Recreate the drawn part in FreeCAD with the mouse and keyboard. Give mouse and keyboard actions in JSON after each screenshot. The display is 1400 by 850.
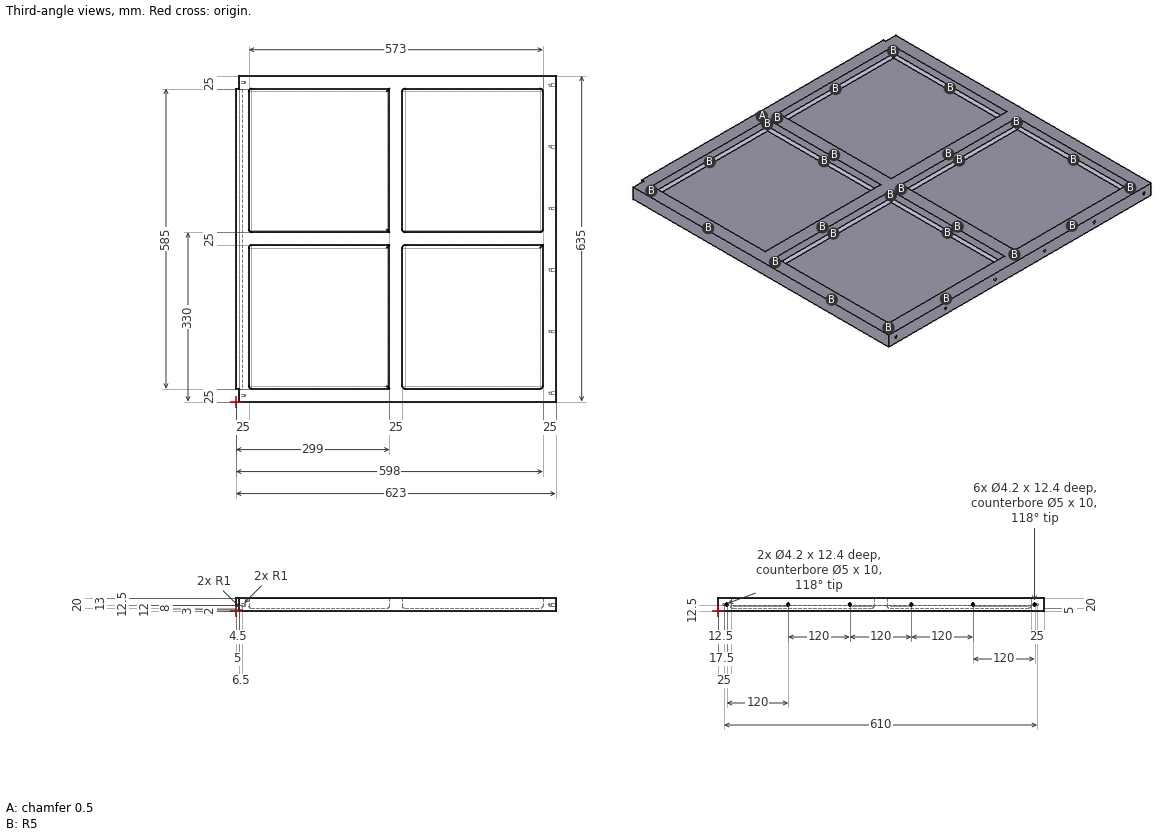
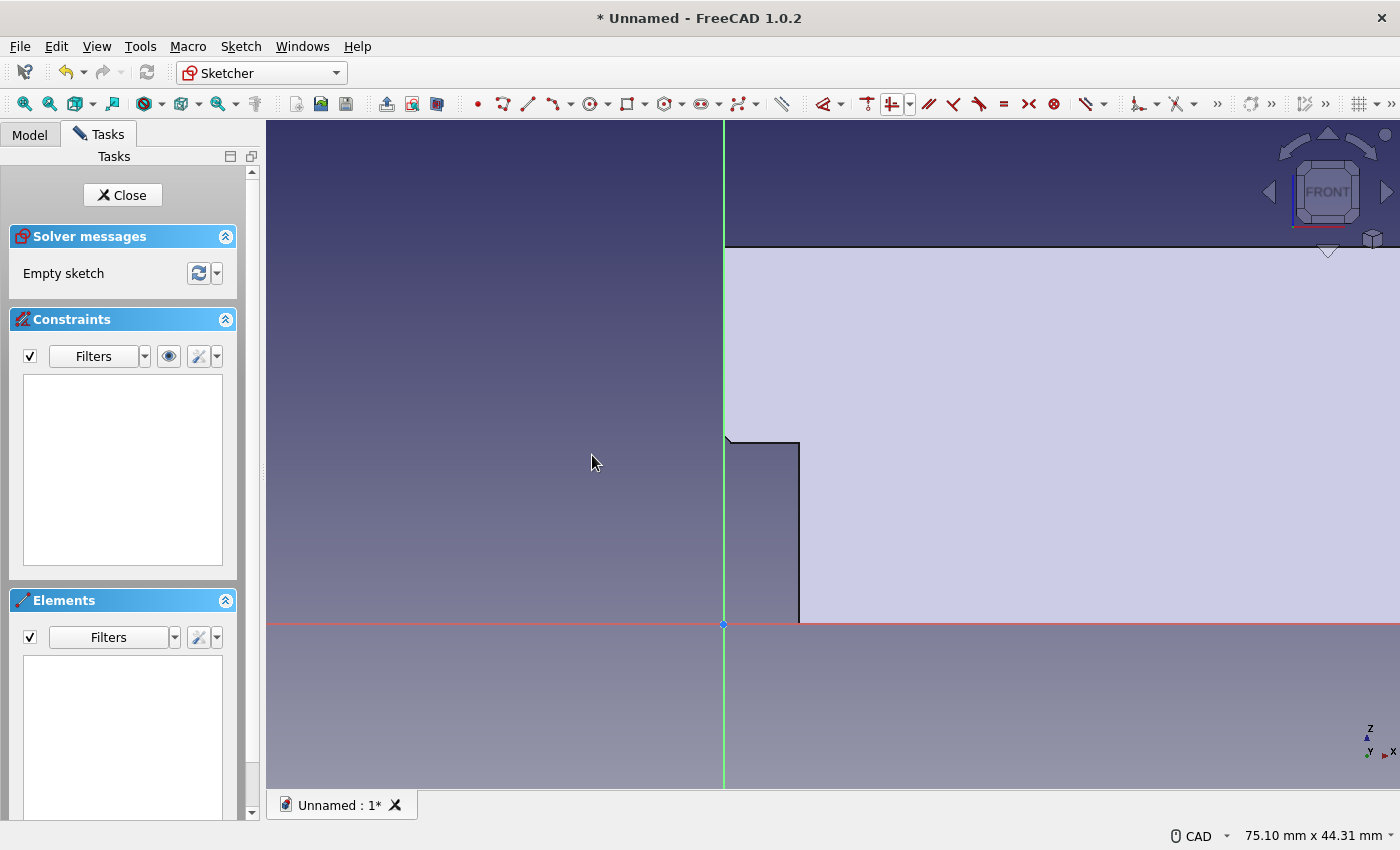
{"action": "left_click", "coordinate": [503, 104]}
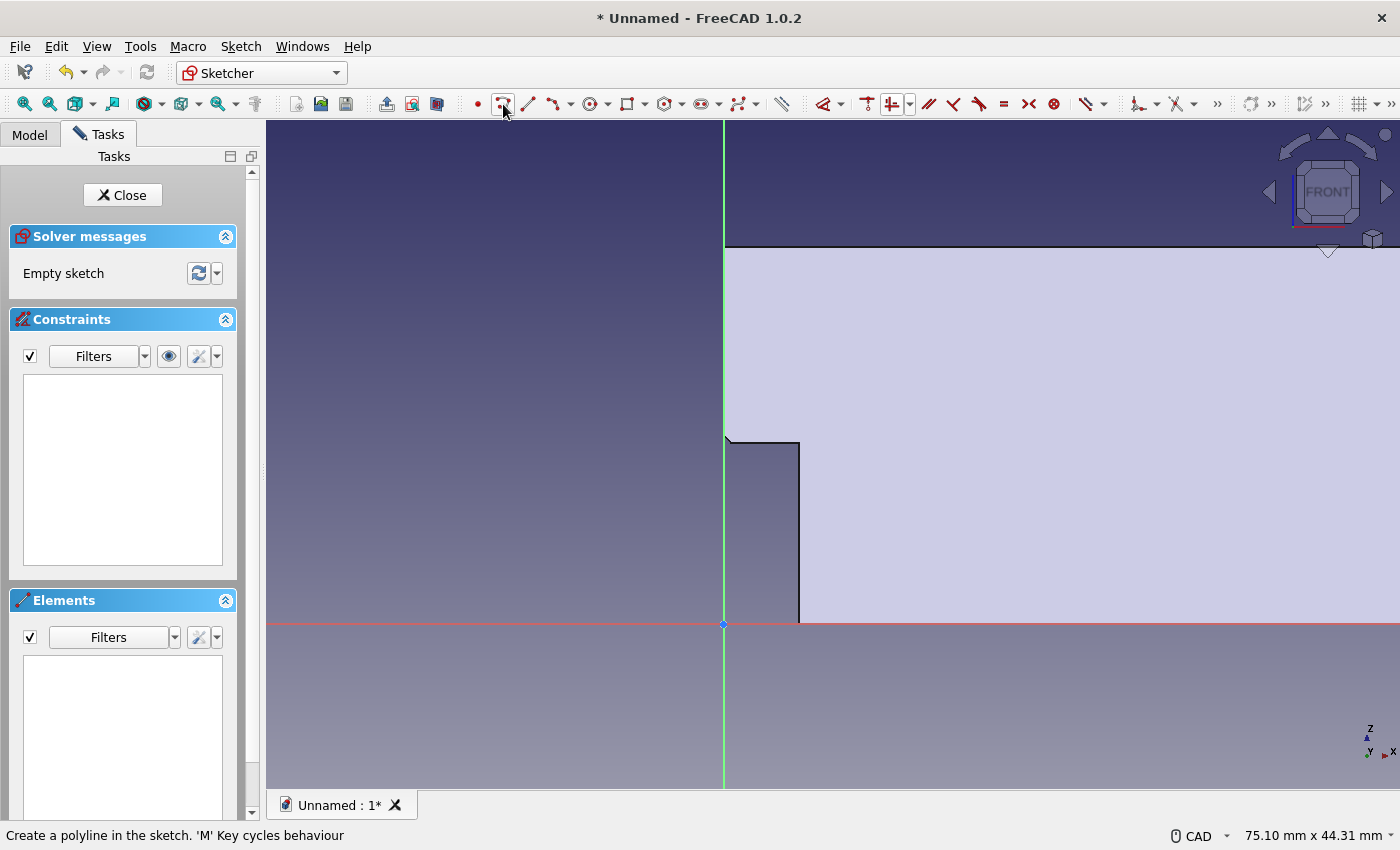
{"action": "scroll", "coordinate": [731, 443], "scroll_direction": "up", "scroll_amount": 4}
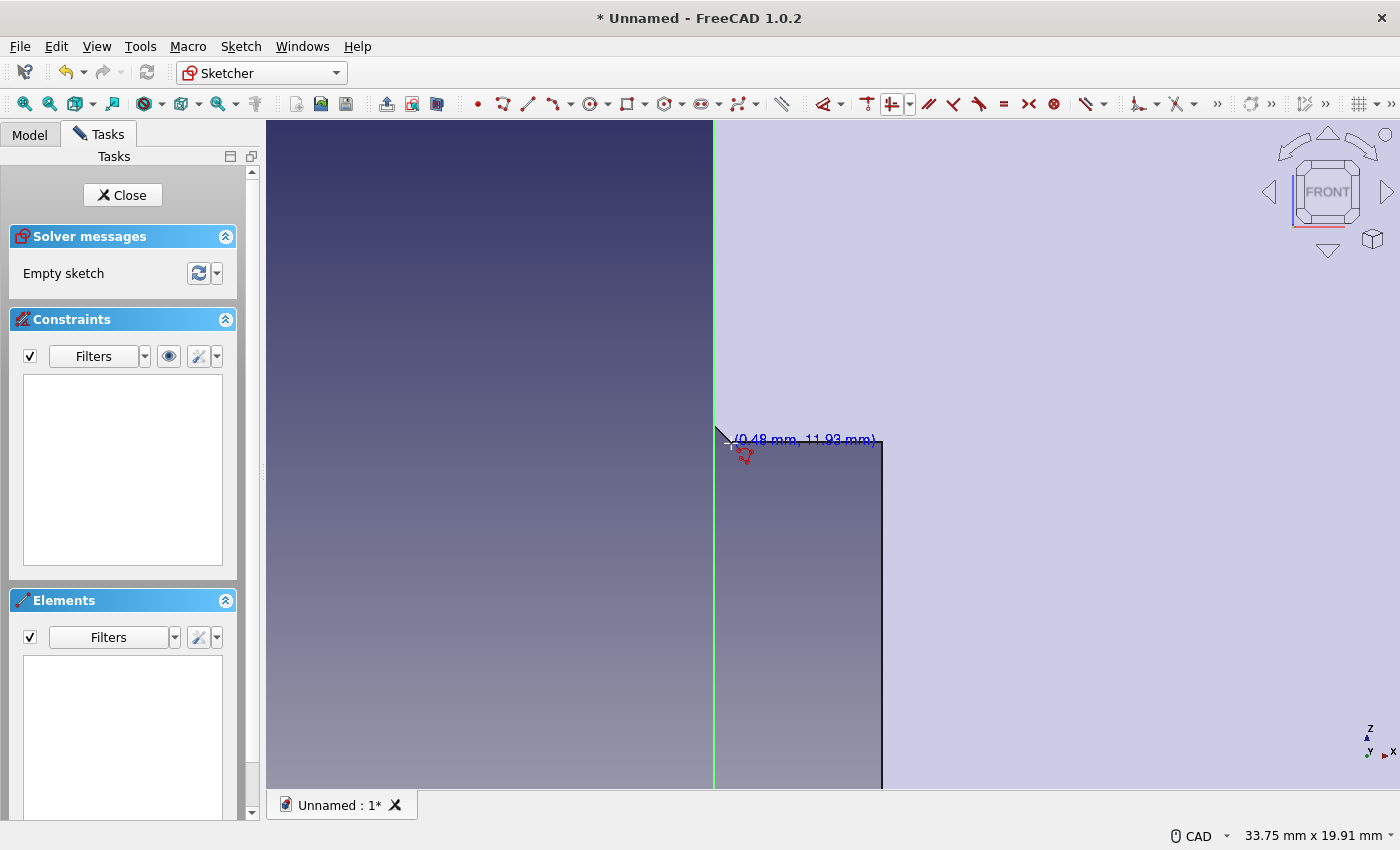
{"action": "left_click", "coordinate": [731, 442]}
{"action": "left_click", "coordinate": [882, 442]}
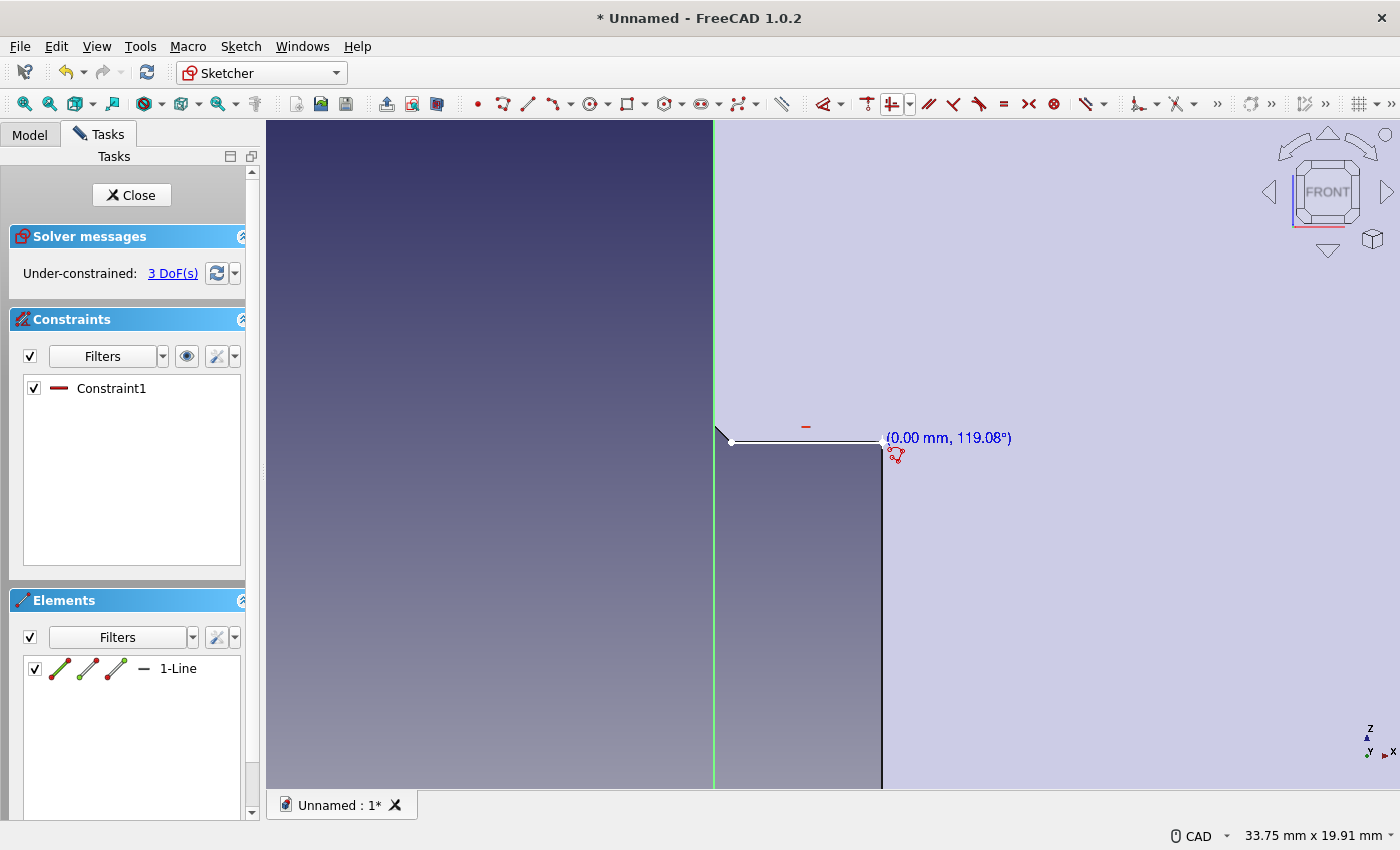
{"action": "scroll", "coordinate": [723, 490], "scroll_direction": "down", "scroll_amount": 3}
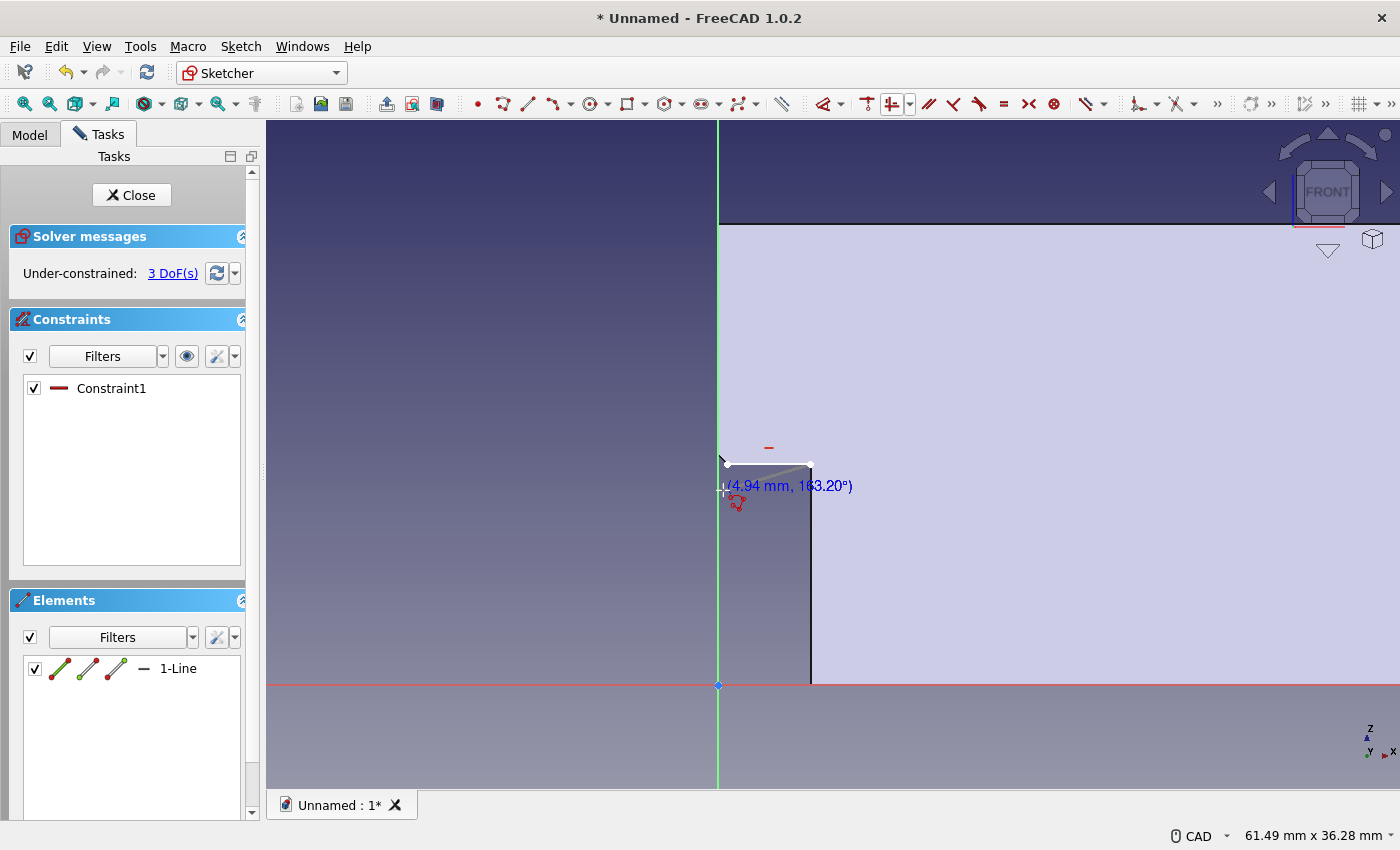
{"action": "left_click", "coordinate": [810, 224]}
{"action": "left_click", "coordinate": [718, 224]}
{"action": "left_click", "coordinate": [727, 455]}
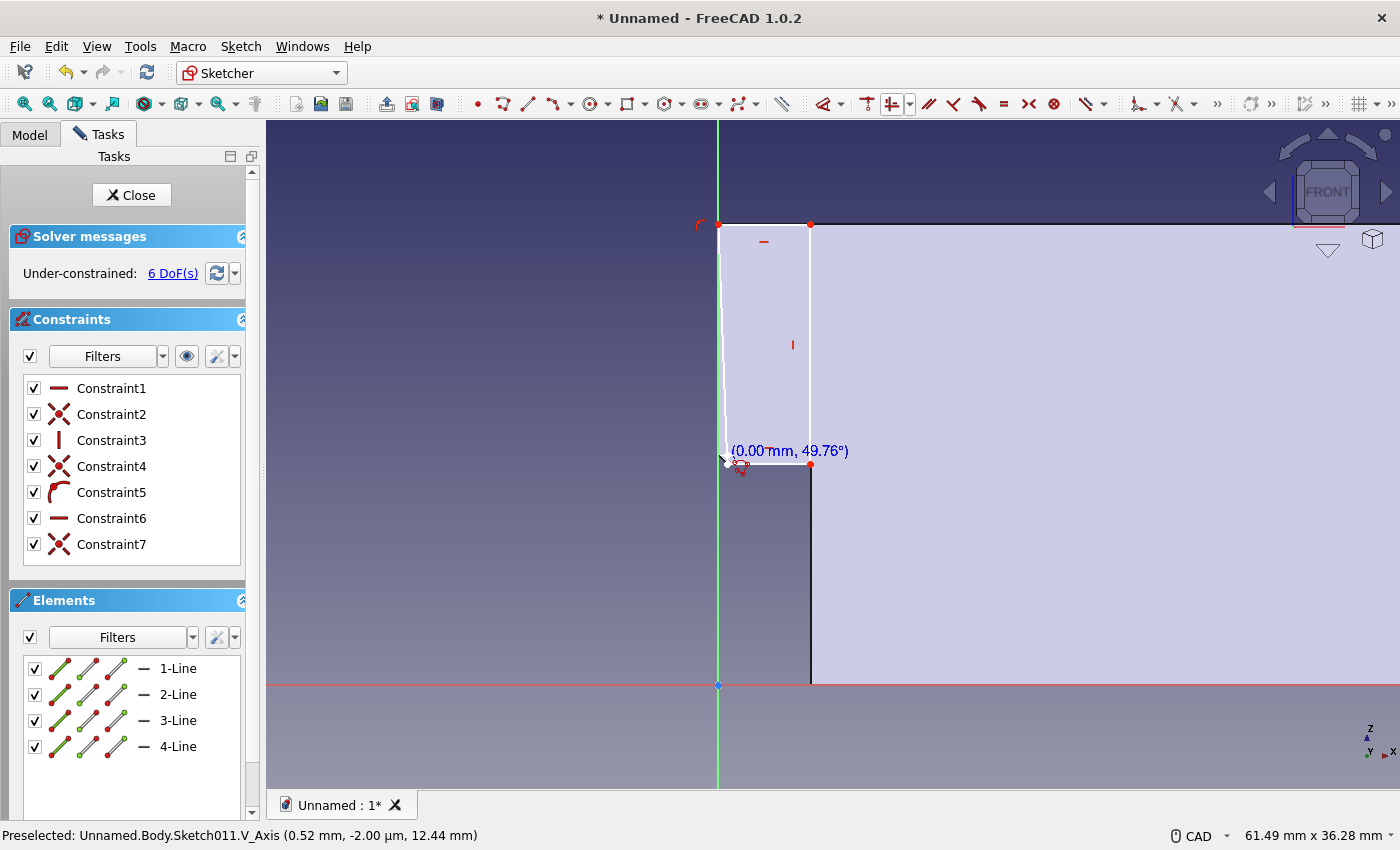
{"action": "scroll", "coordinate": [728, 464], "scroll_direction": "up", "scroll_amount": 3}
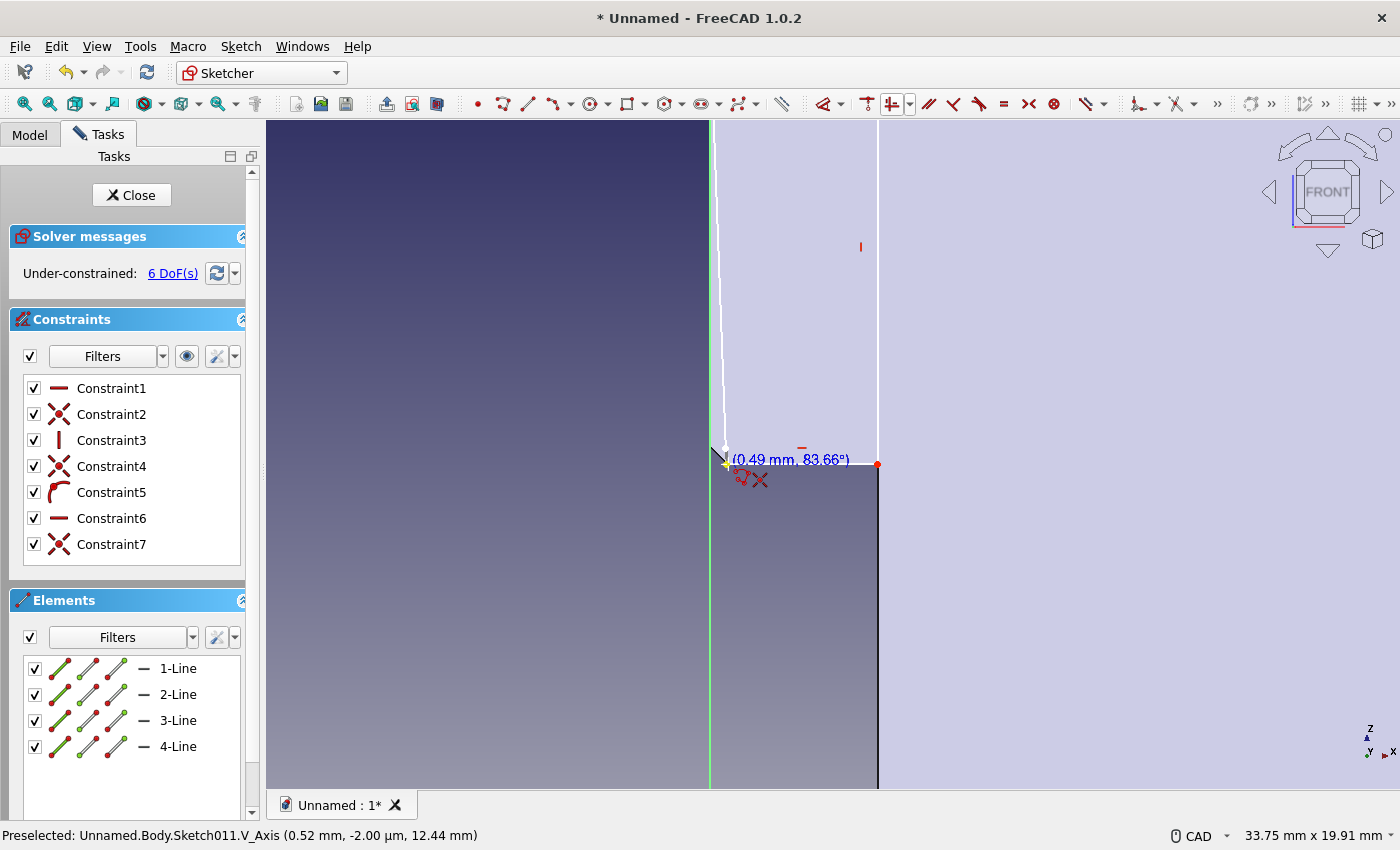
{"action": "left_click", "coordinate": [727, 464]}
{"action": "key", "text": "Escape"}
{"action": "key", "text": "Escape"}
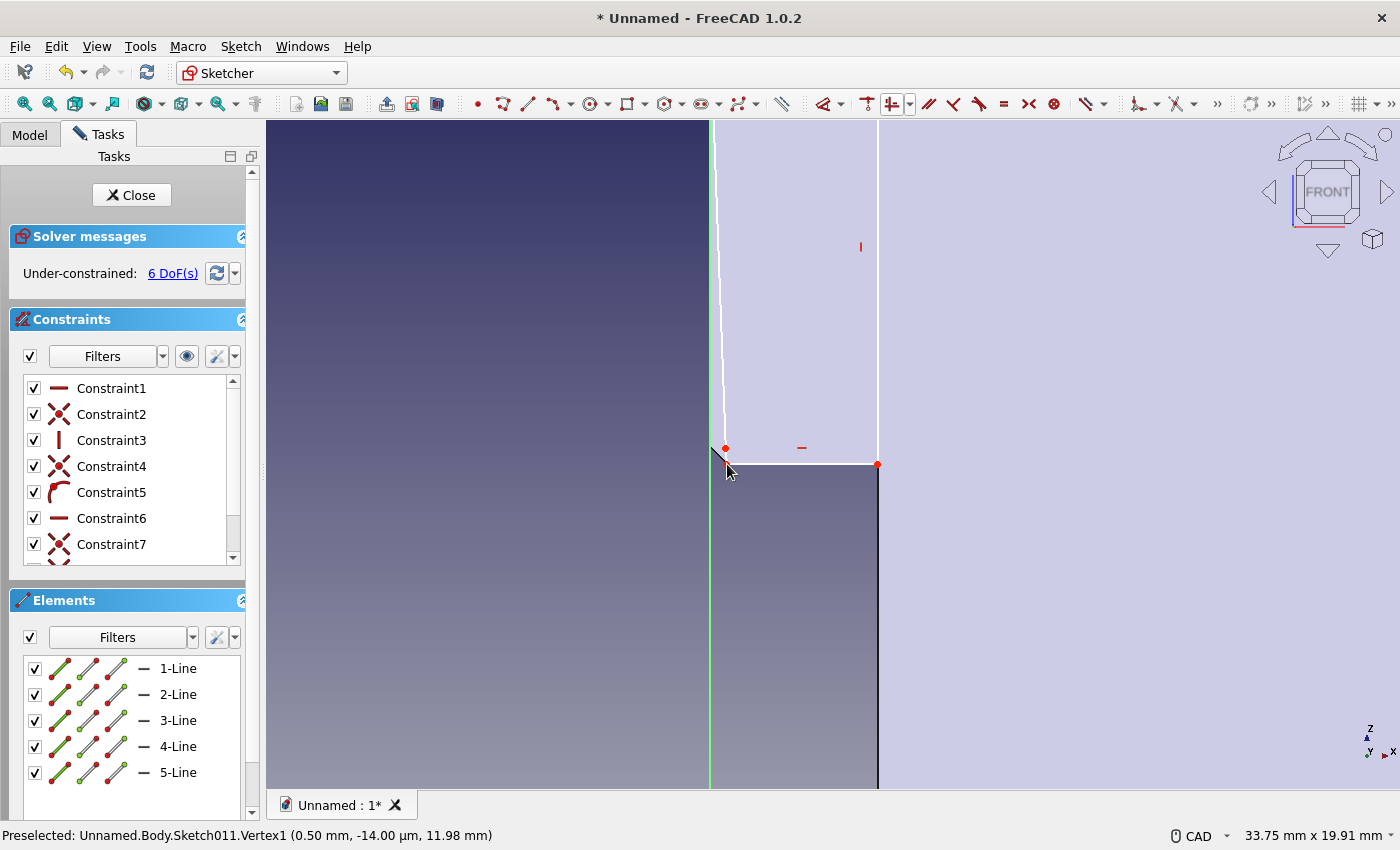
{"action": "scroll", "coordinate": [721, 323], "scroll_direction": "up", "scroll_amount": 2}